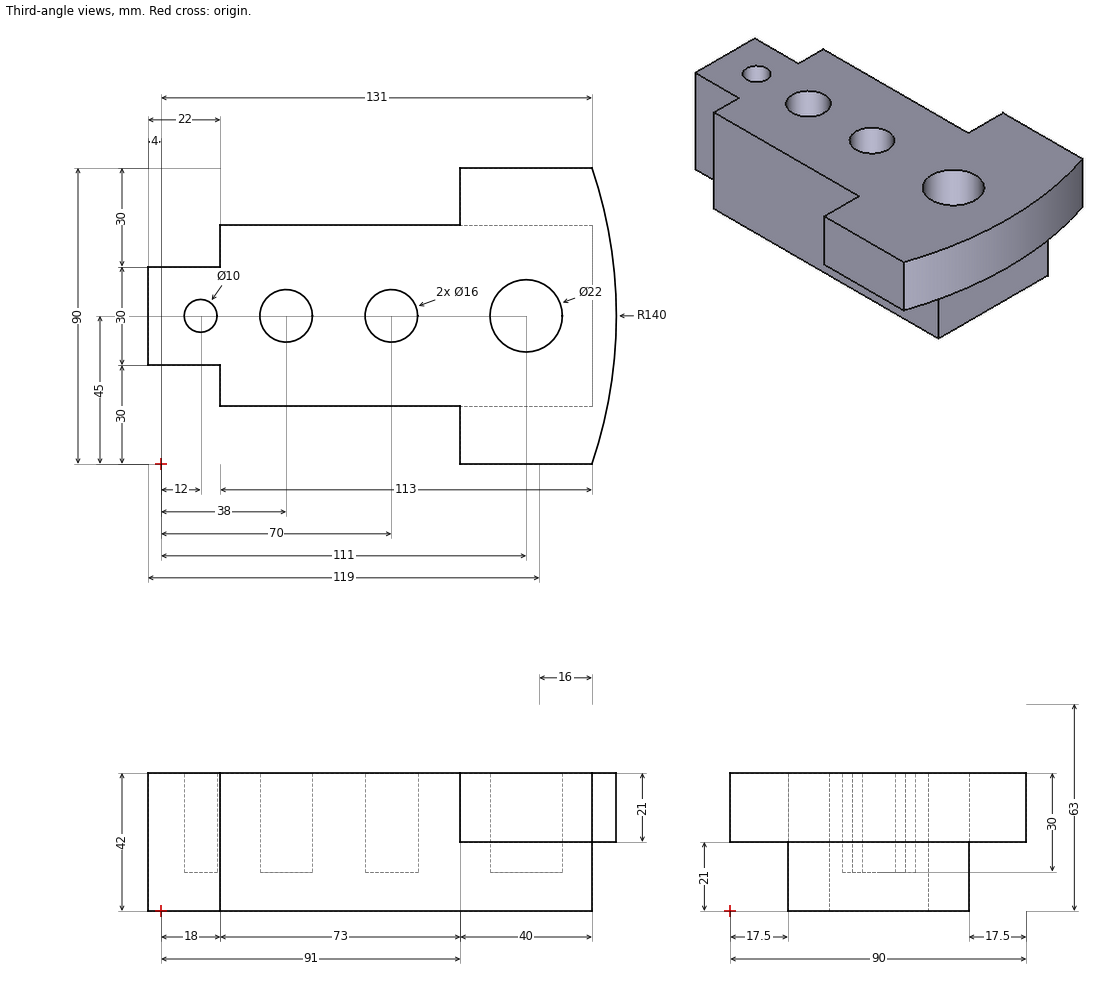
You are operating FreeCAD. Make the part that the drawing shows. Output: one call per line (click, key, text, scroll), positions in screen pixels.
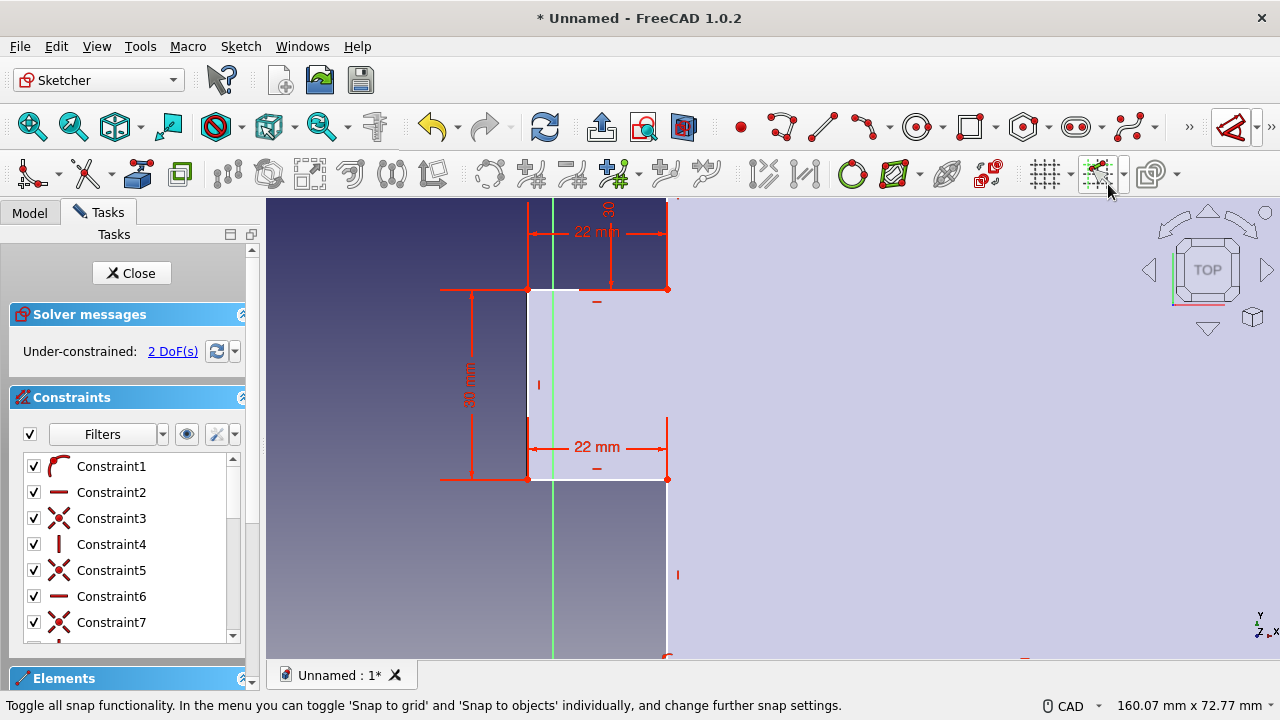
scroll(528, 290, up, 3)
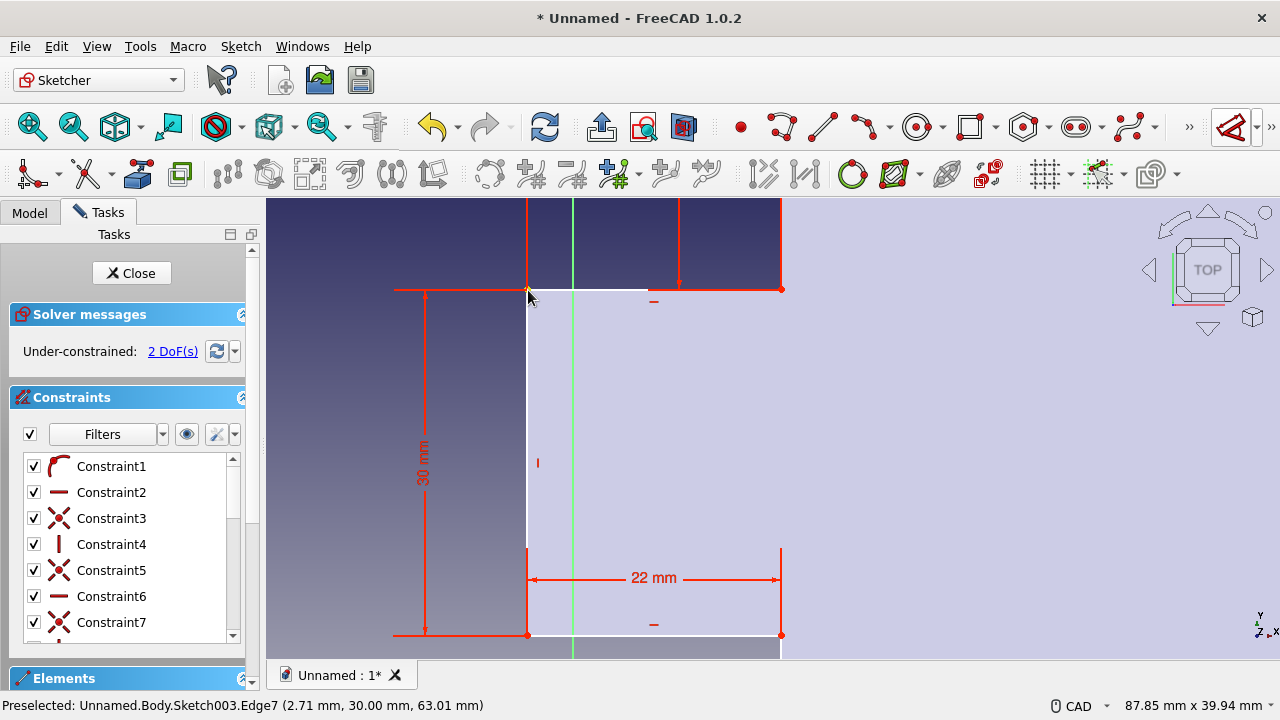
click(527, 290)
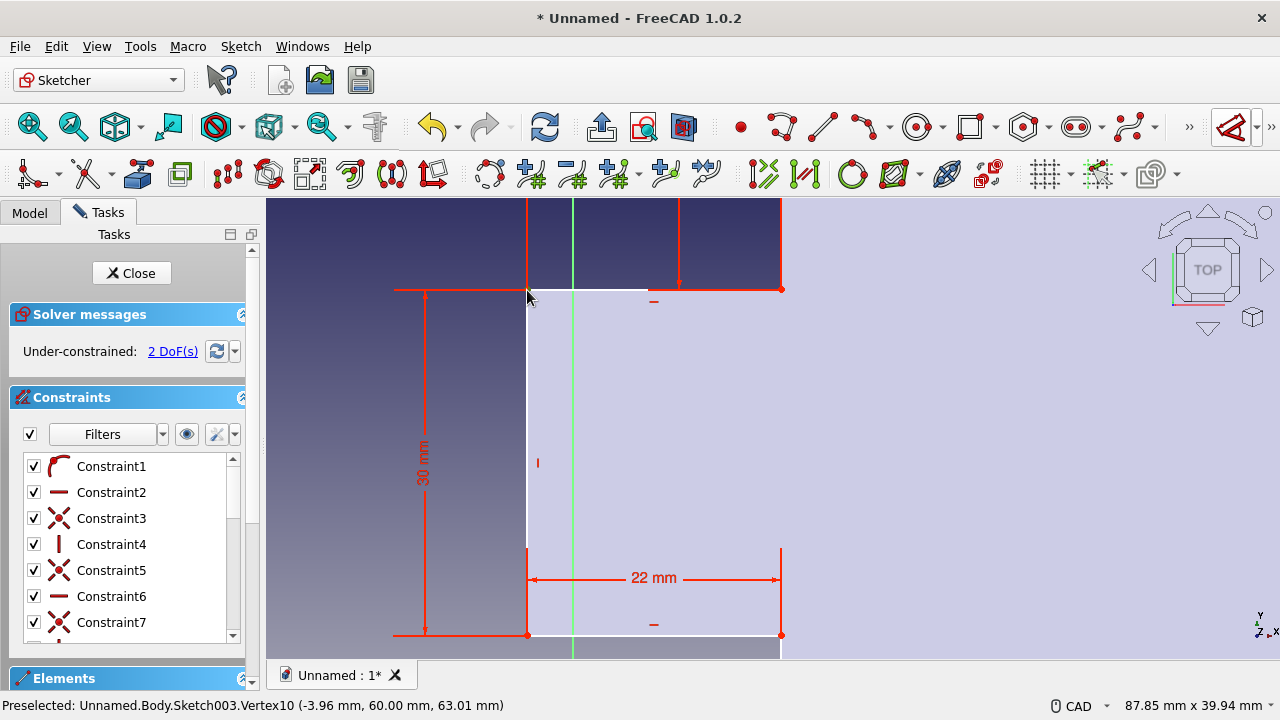
click(1256, 128)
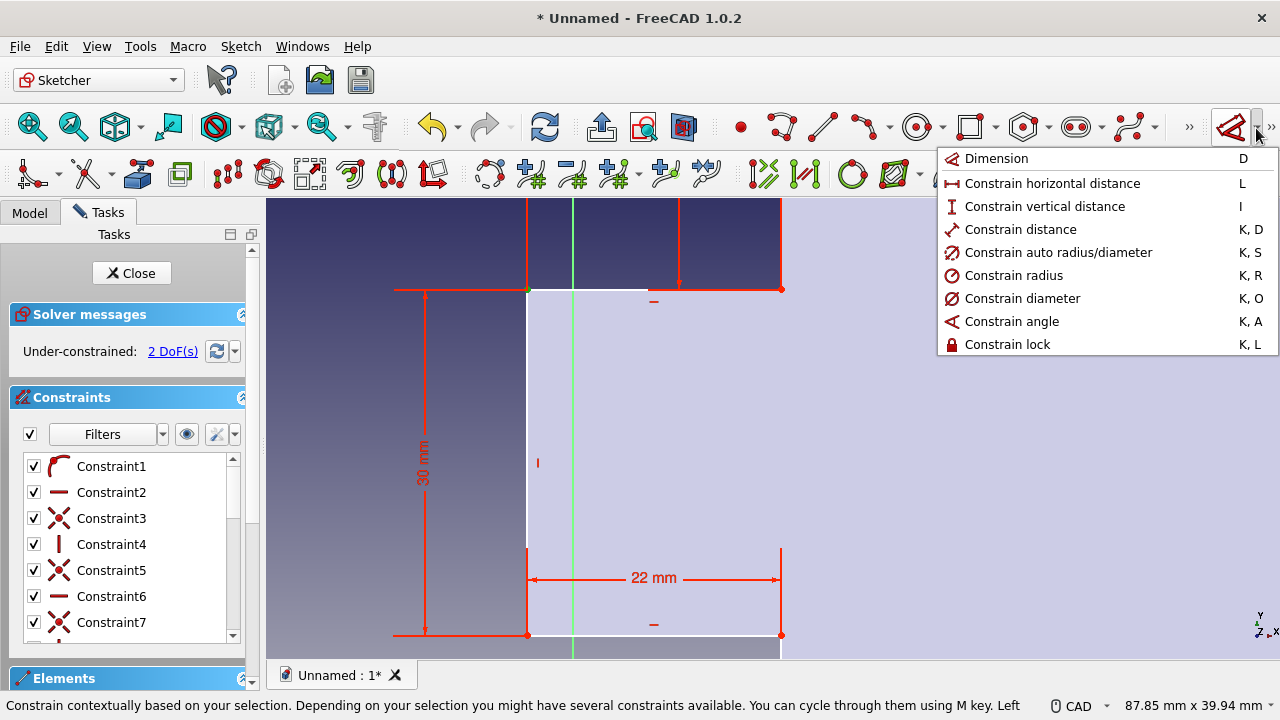
click(1108, 184)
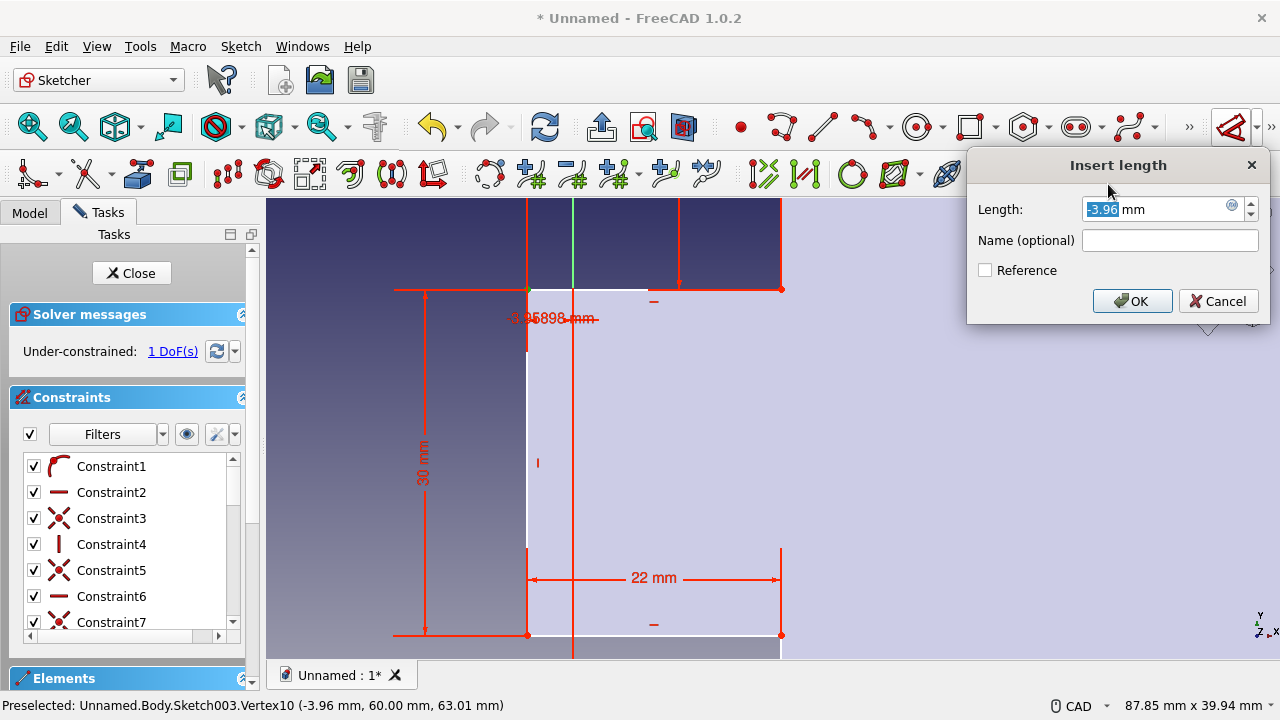
text(-4)
key(Return)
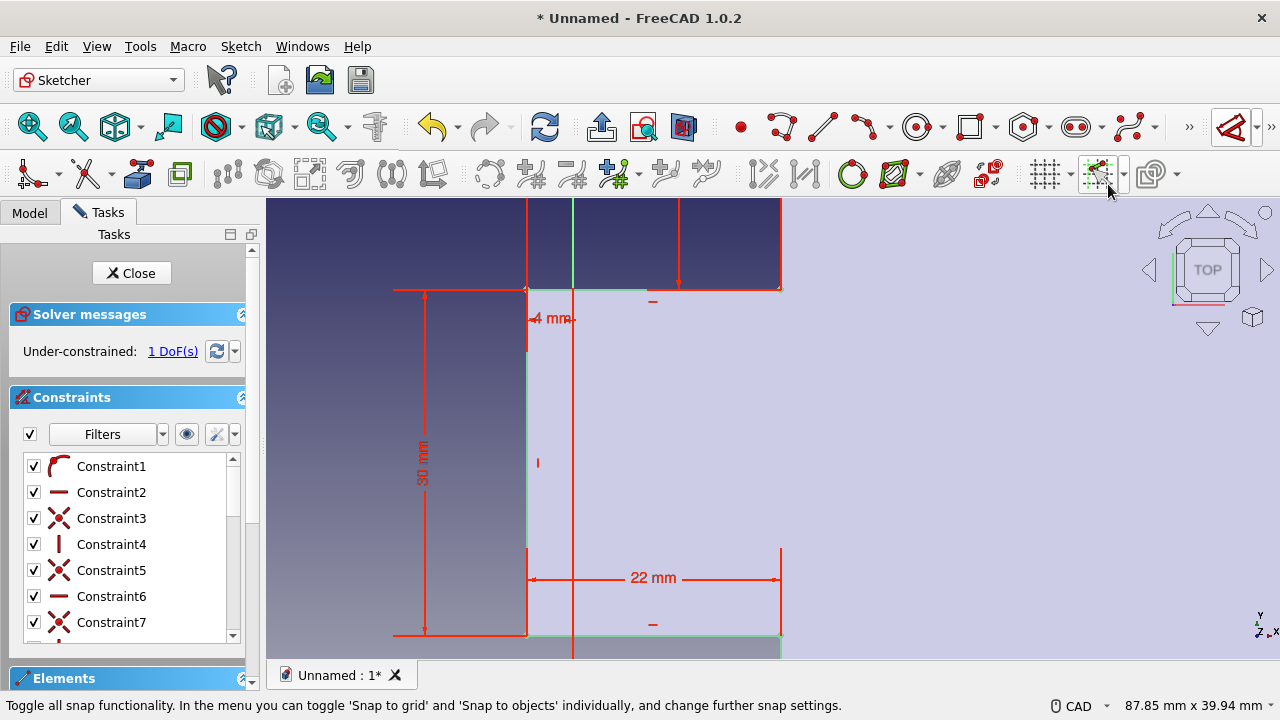
scroll(445, 414, down, 6)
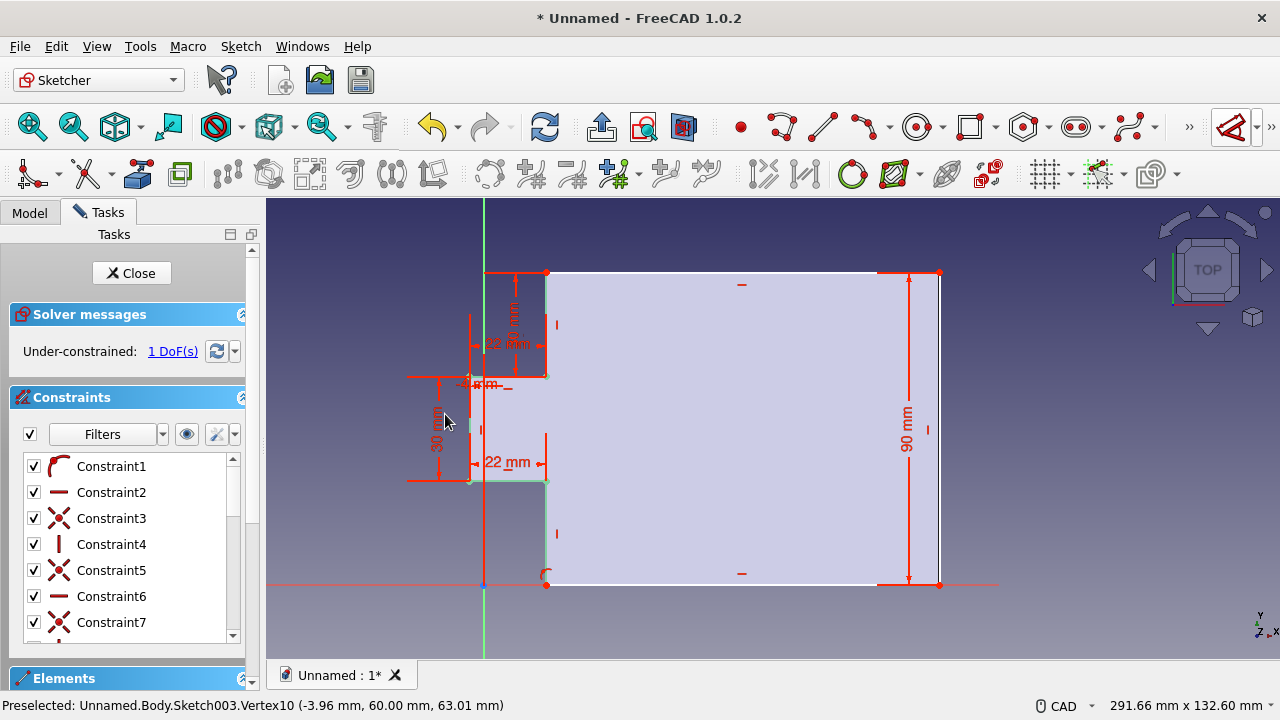
click(664, 585)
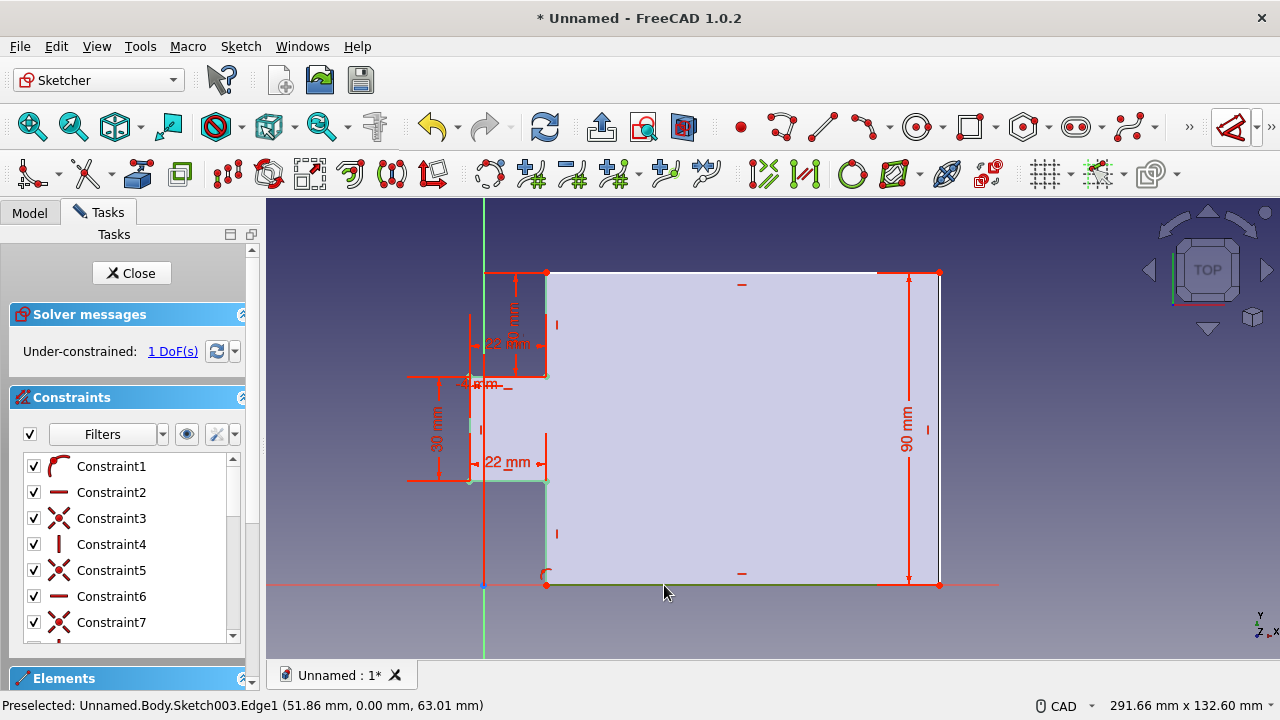
key(l)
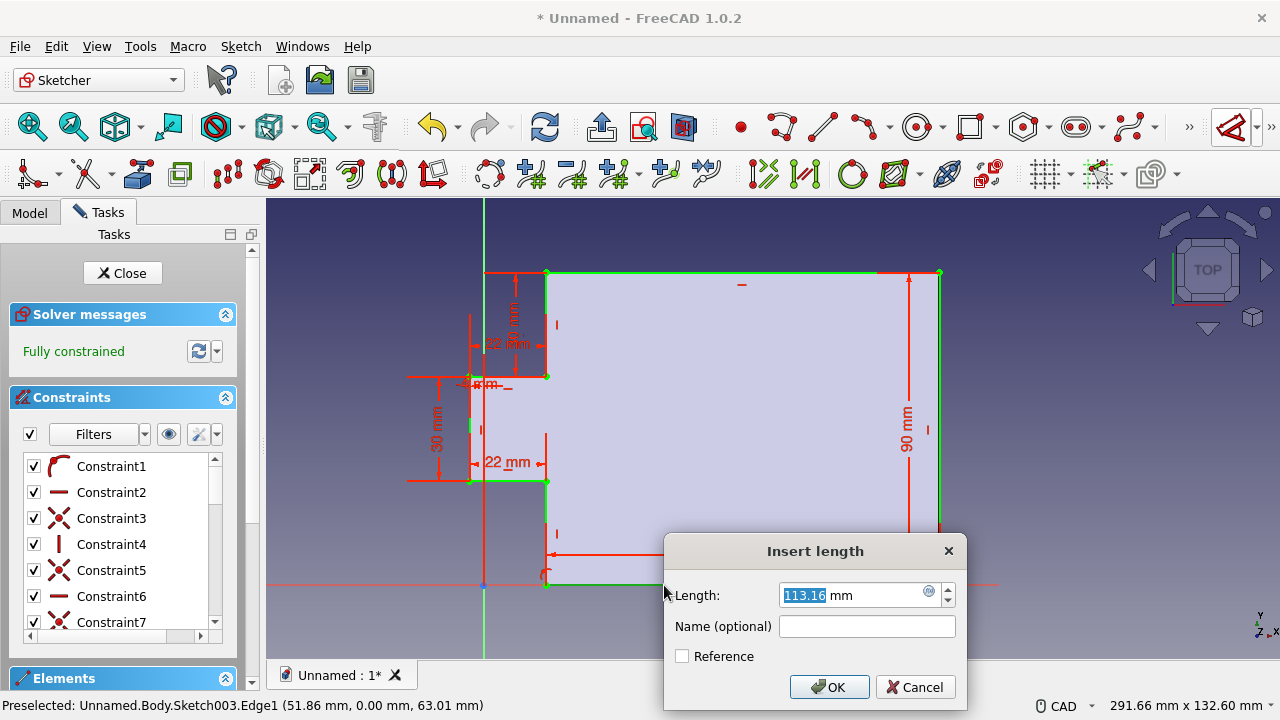
text(113)
key(Return)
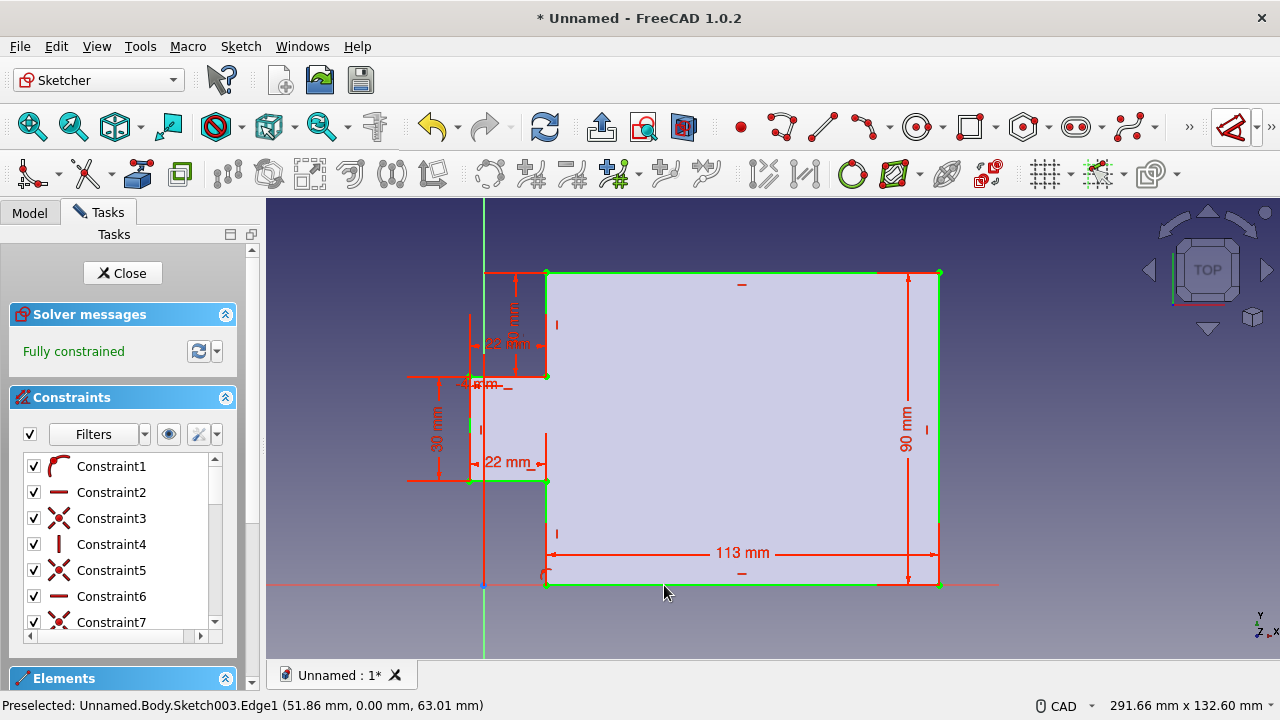
click(123, 273)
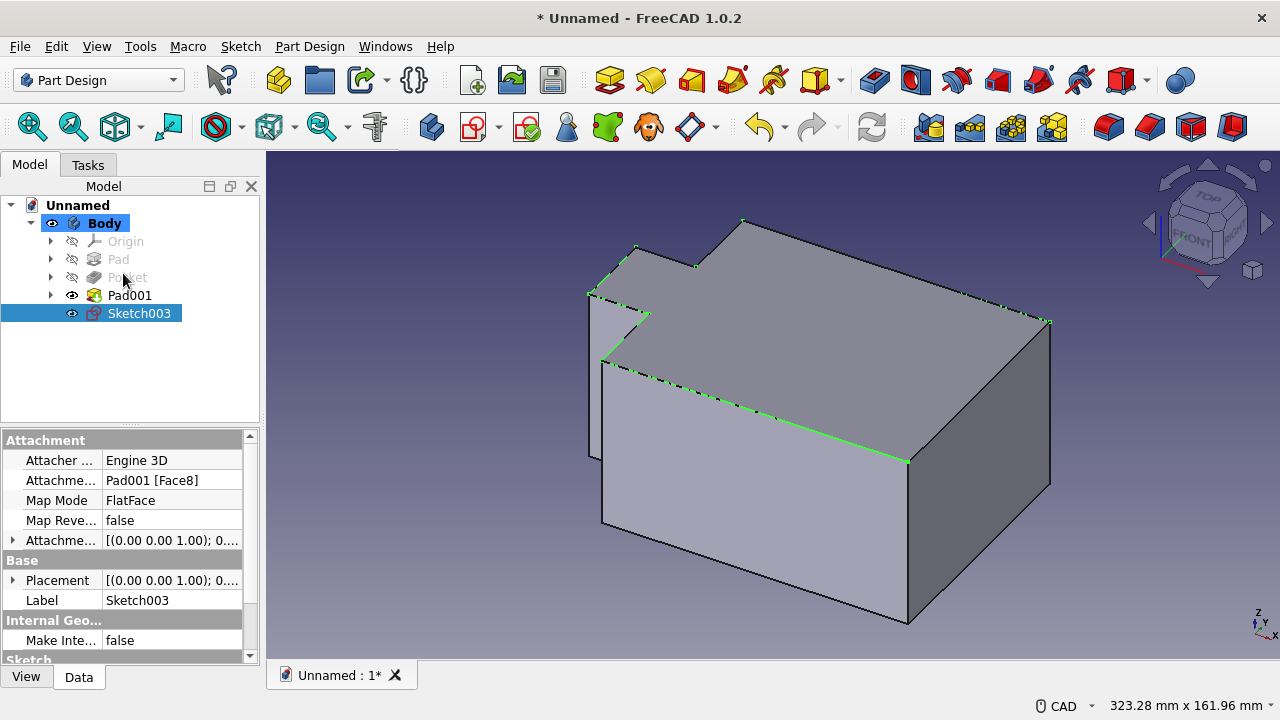
click(875, 80)